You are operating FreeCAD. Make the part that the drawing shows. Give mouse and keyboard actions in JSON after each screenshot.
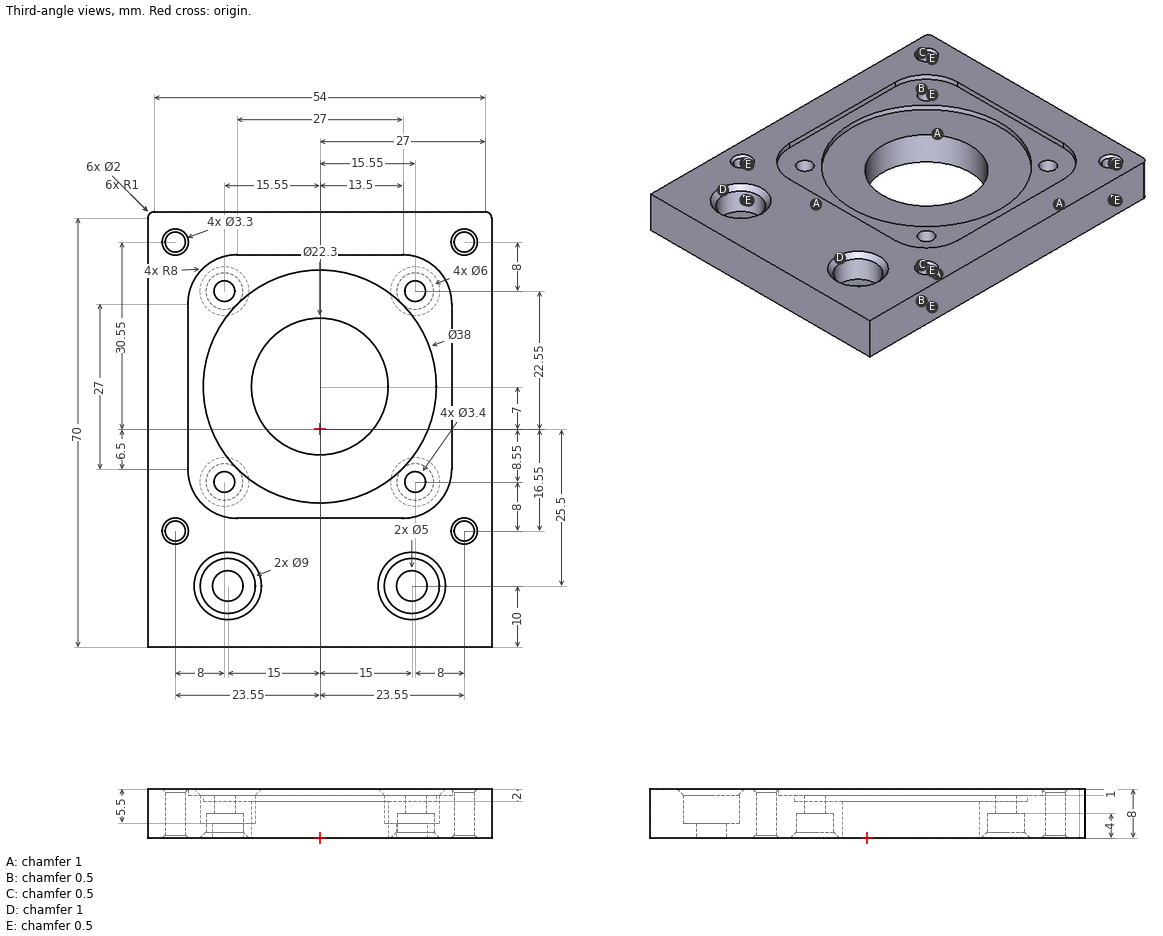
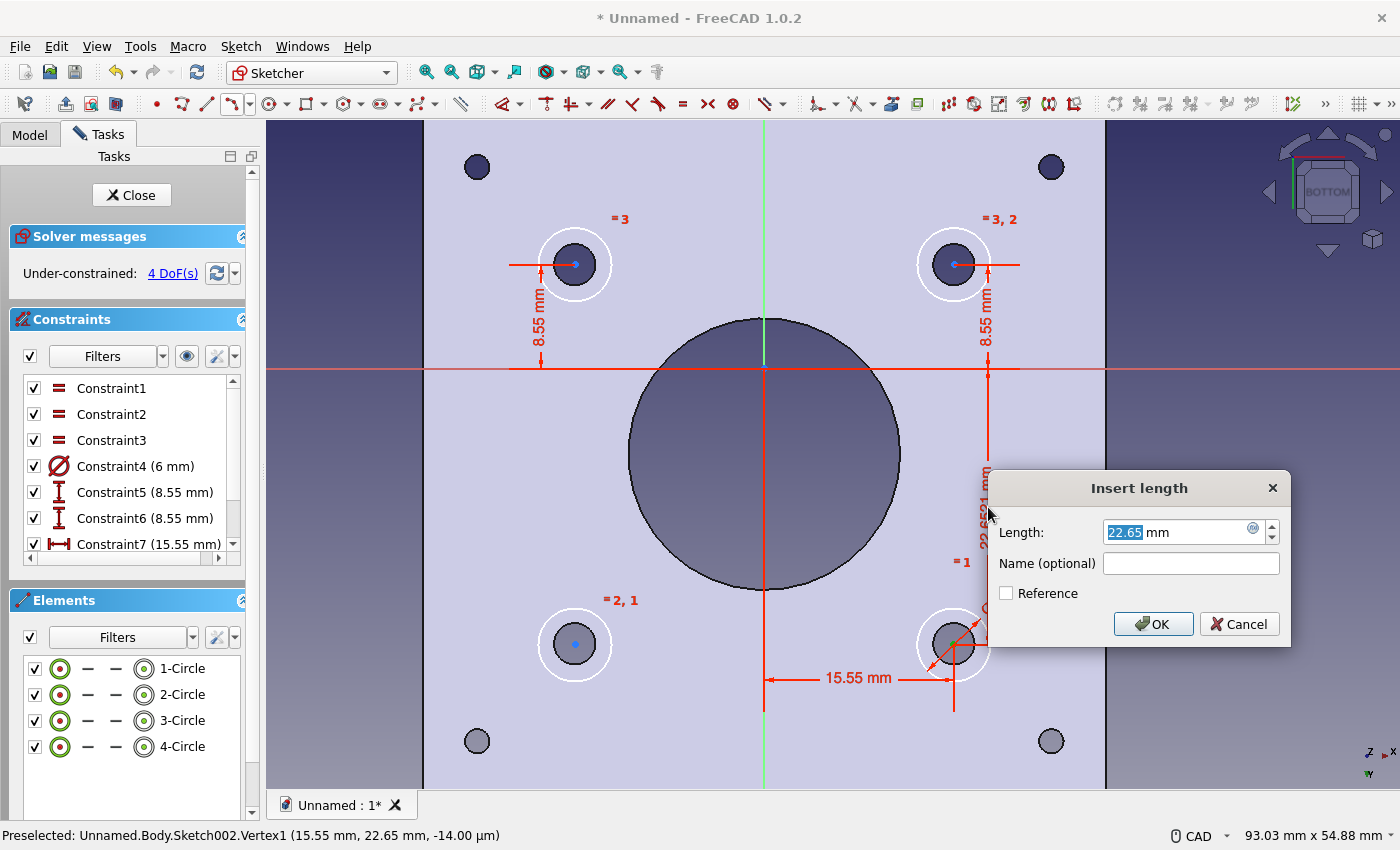
{"action": "type", "text": "22.55"}
{"action": "key", "text": "Return"}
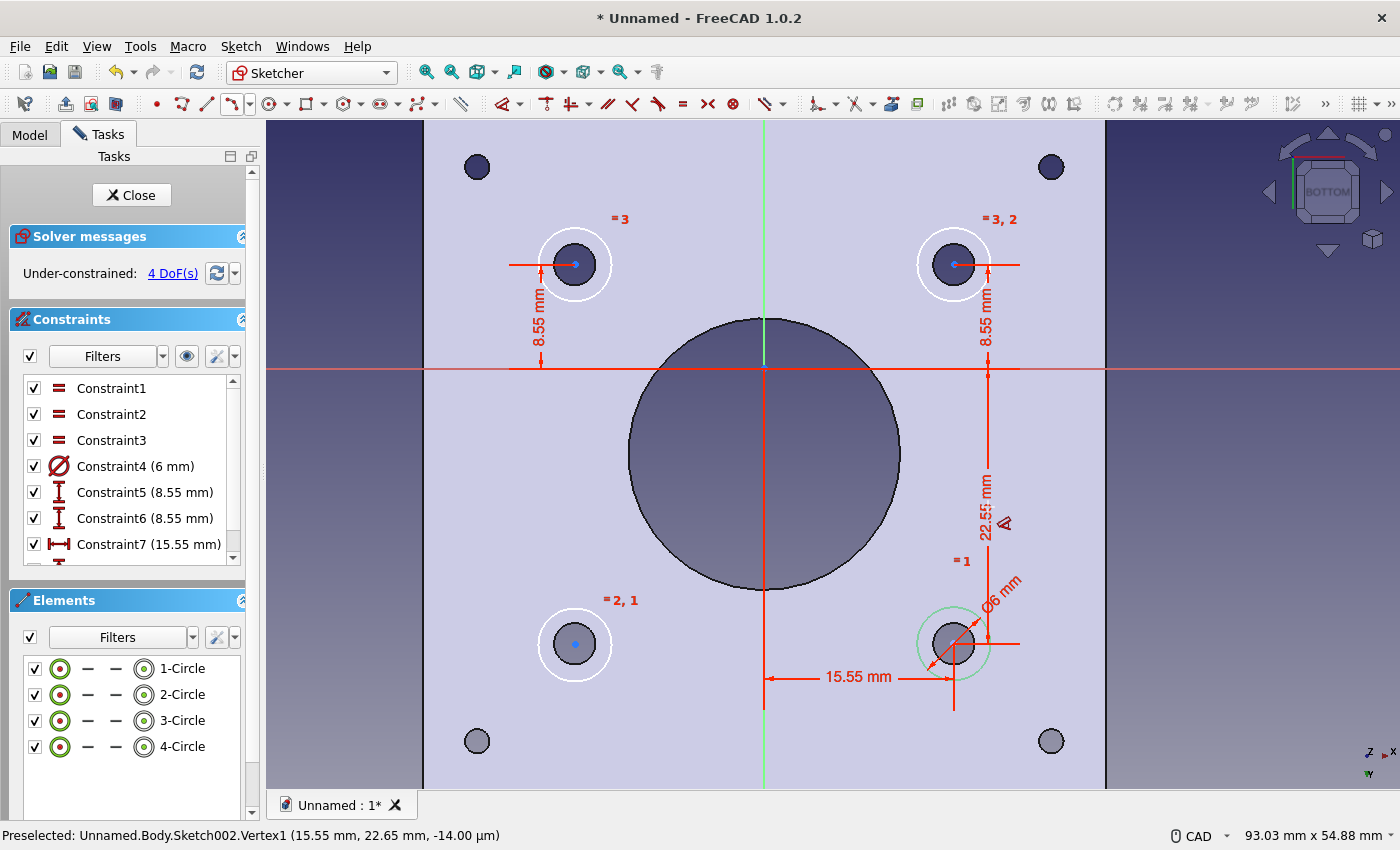
{"action": "left_click", "coordinate": [575, 645]}
{"action": "left_click", "coordinate": [670, 679]}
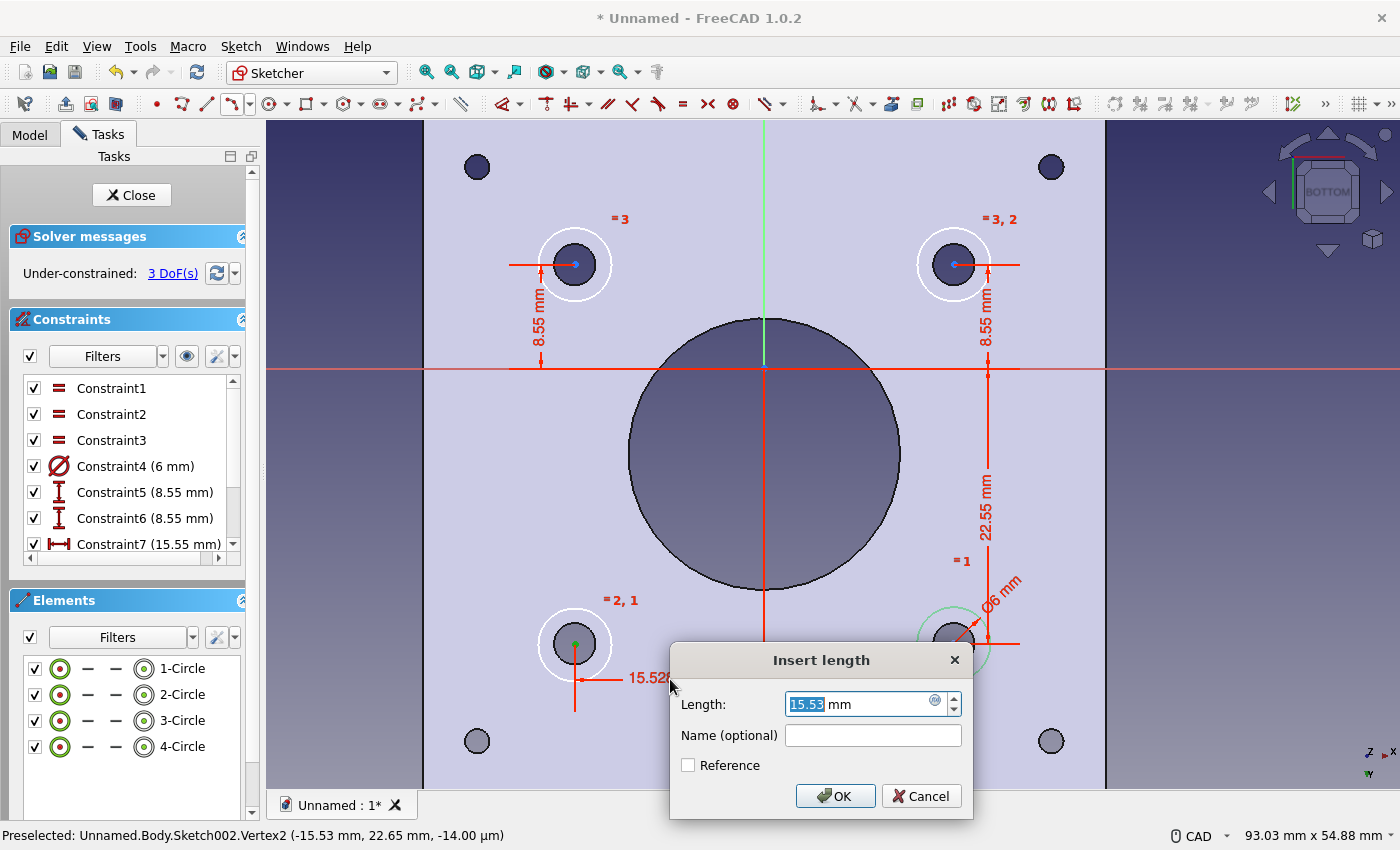
{"action": "type", "text": "15.55"}
{"action": "key", "text": "Return"}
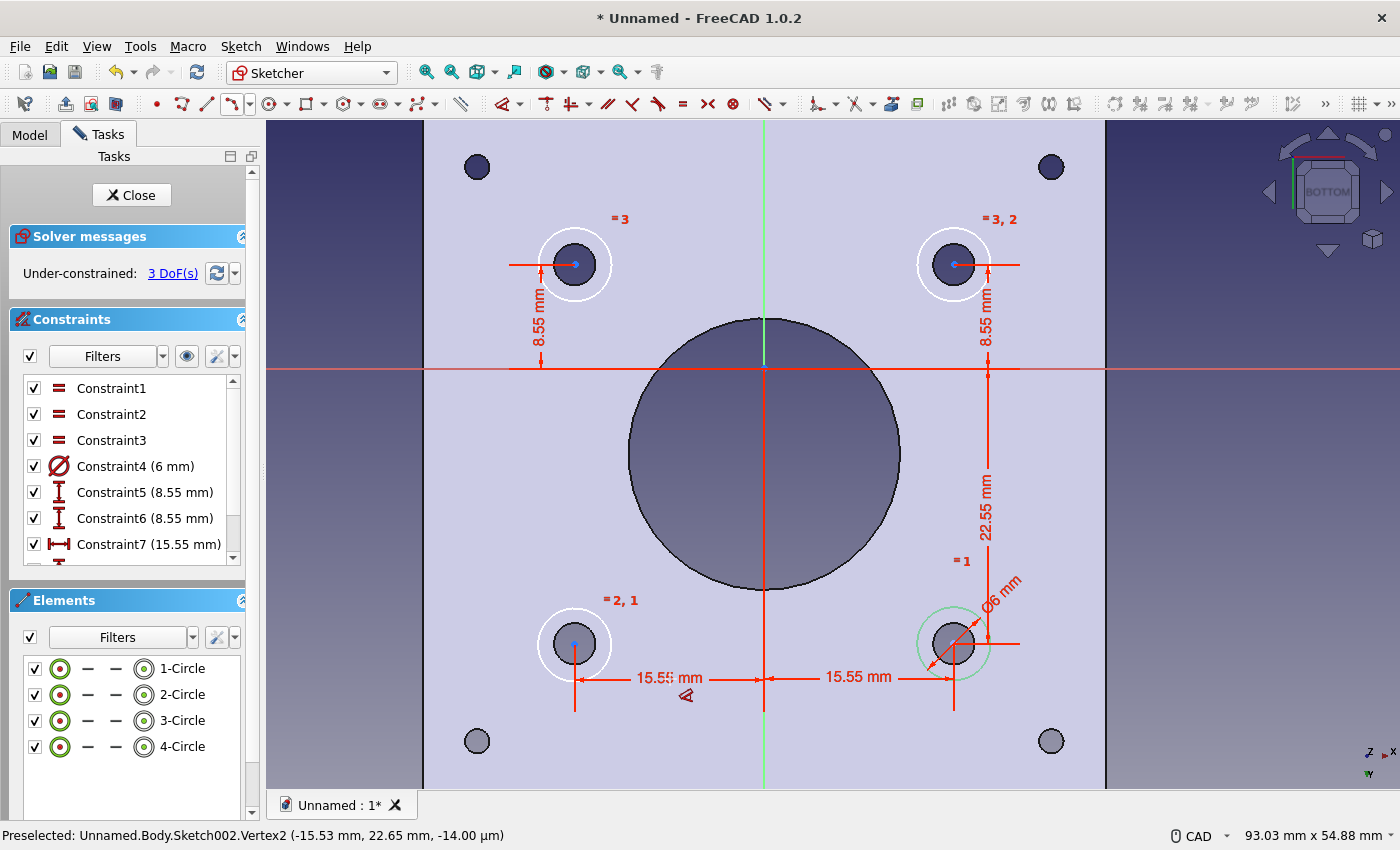
{"action": "left_click", "coordinate": [575, 645]}
{"action": "left_click", "coordinate": [541, 507]}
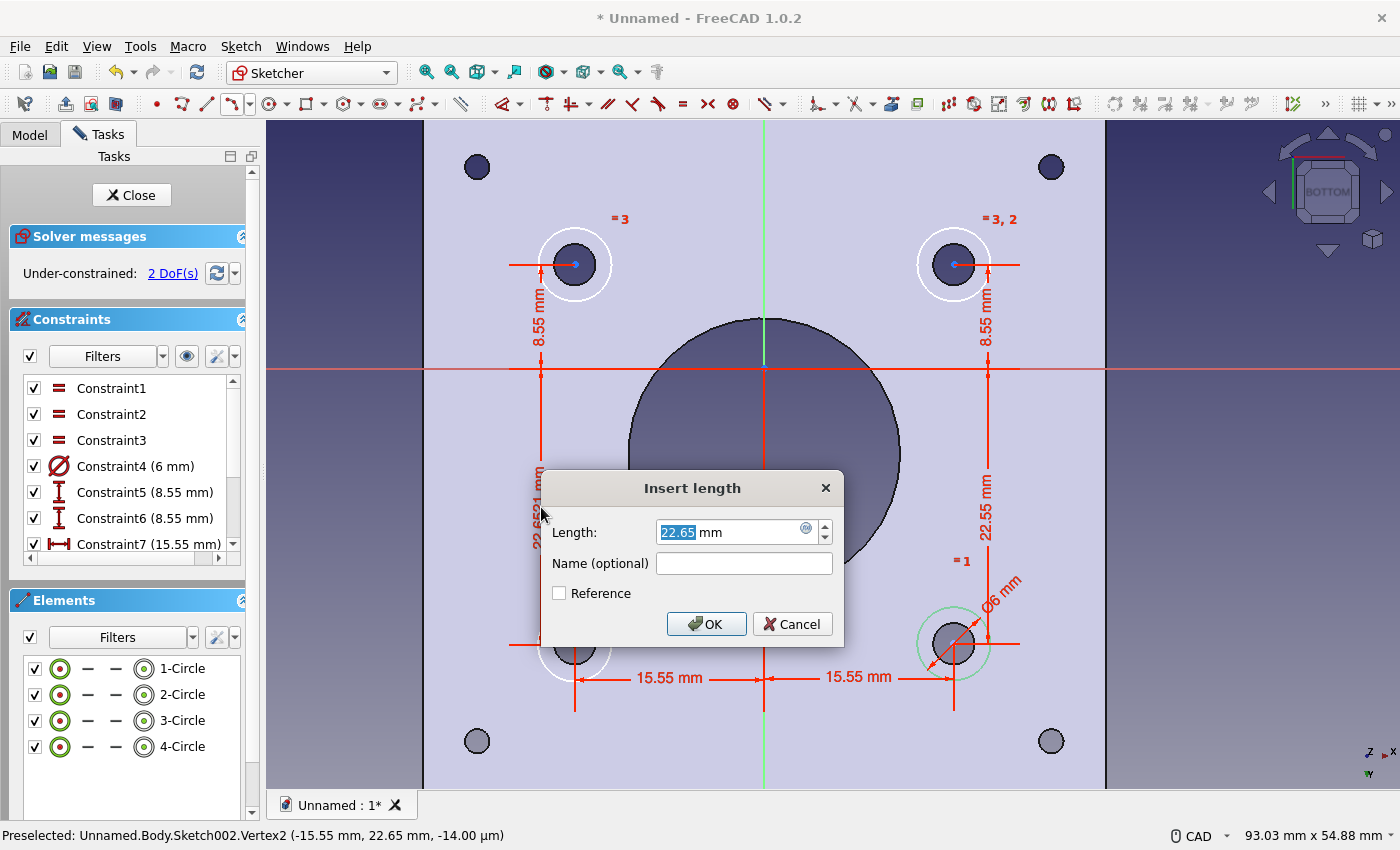
{"action": "type", "text": "22.55"}
{"action": "key", "text": "Return"}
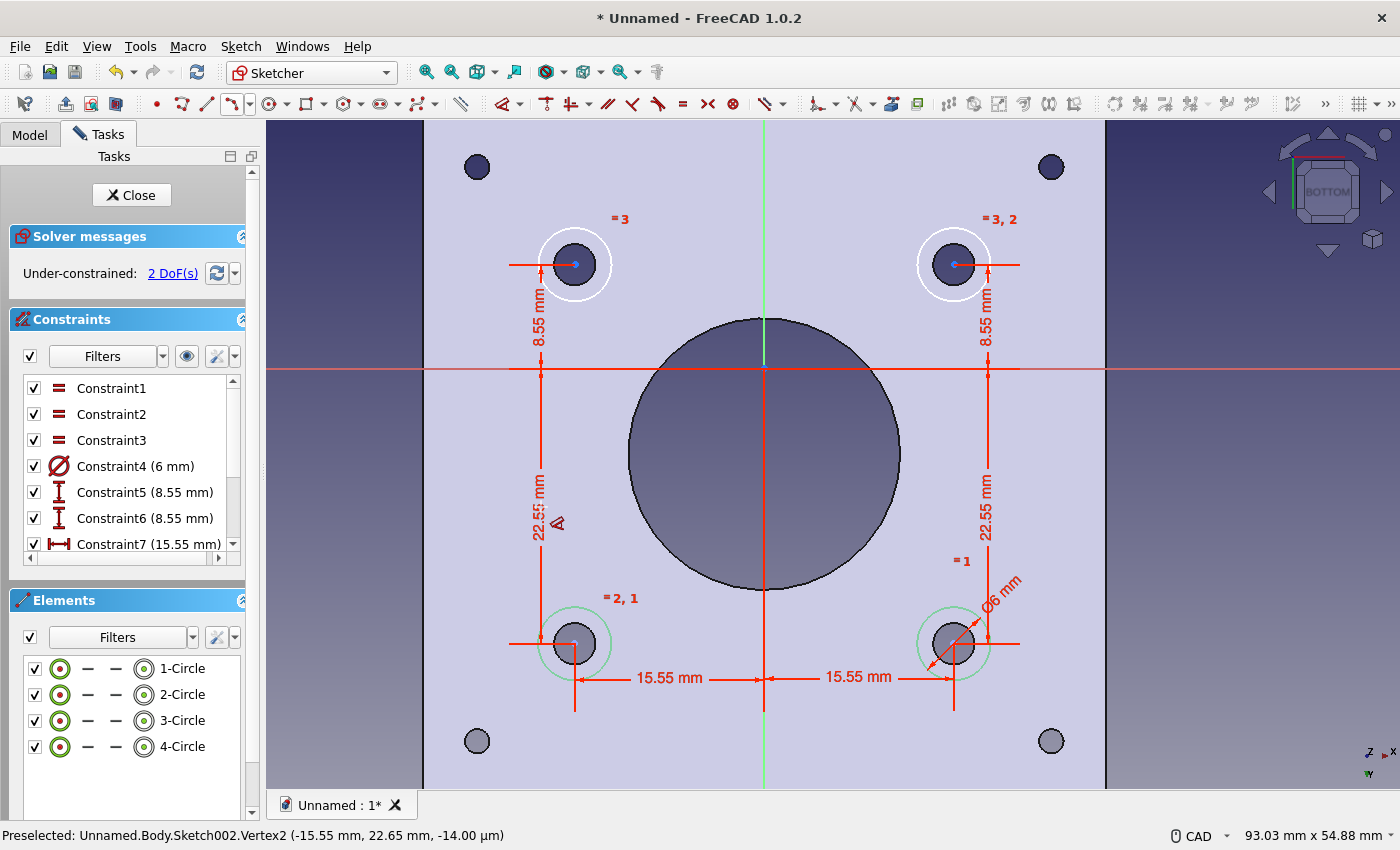
{"action": "left_click", "coordinate": [954, 265]}
{"action": "left_click", "coordinate": [859, 231]}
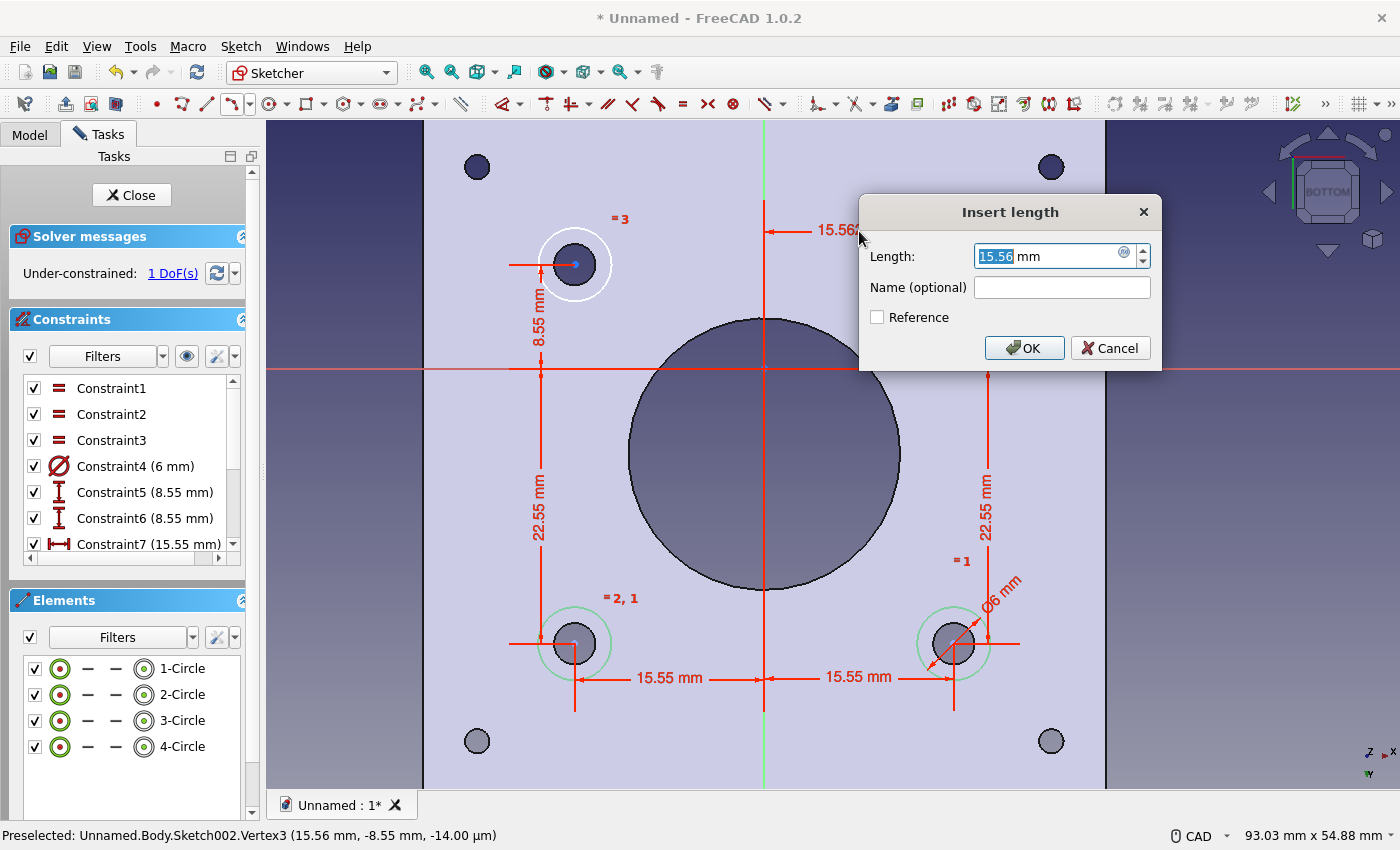
{"action": "type", "text": "15.55"}
{"action": "key", "text": "Return"}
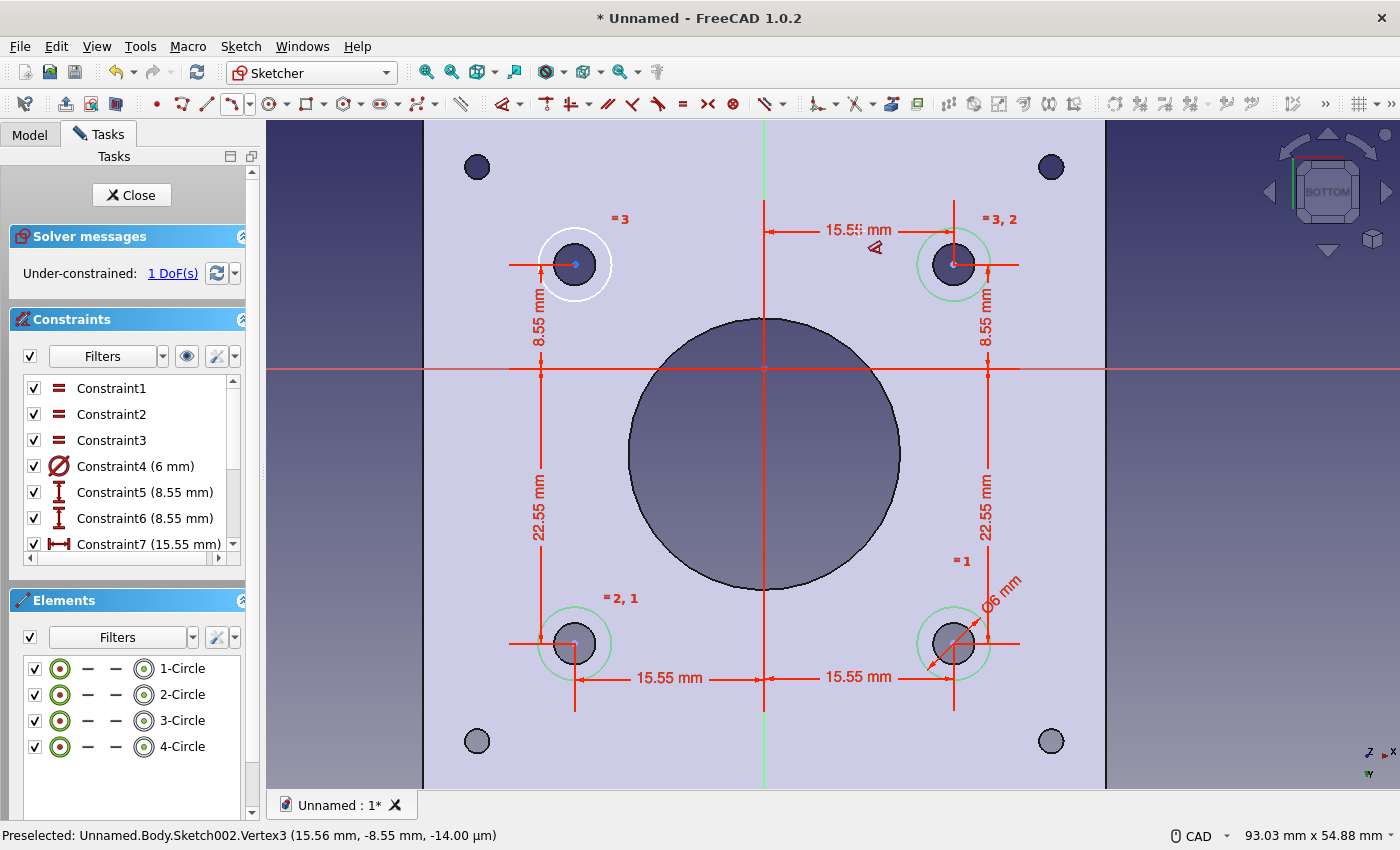
{"action": "left_click", "coordinate": [575, 265]}
{"action": "left_click", "coordinate": [670, 231]}